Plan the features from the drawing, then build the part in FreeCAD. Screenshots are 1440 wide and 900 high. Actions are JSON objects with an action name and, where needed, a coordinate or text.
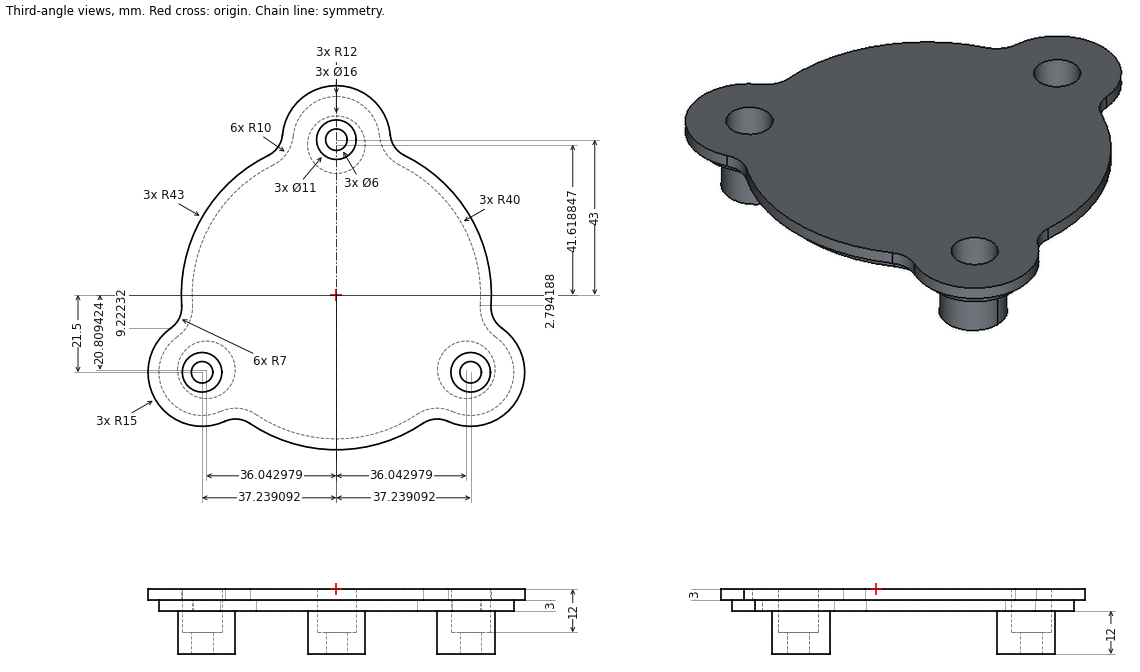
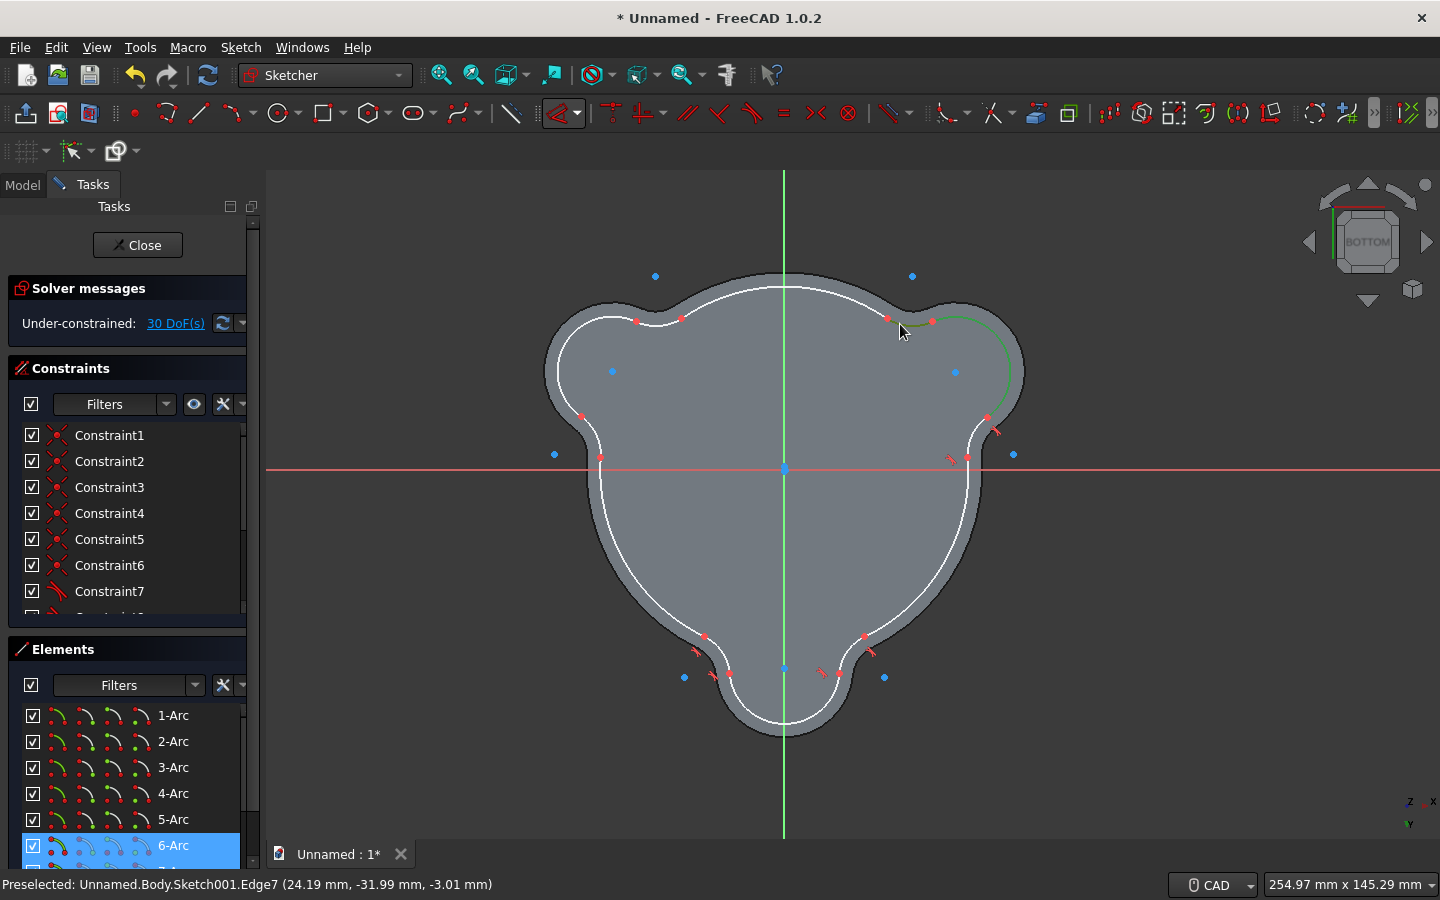
{"action": "left_click", "coordinate": [752, 114]}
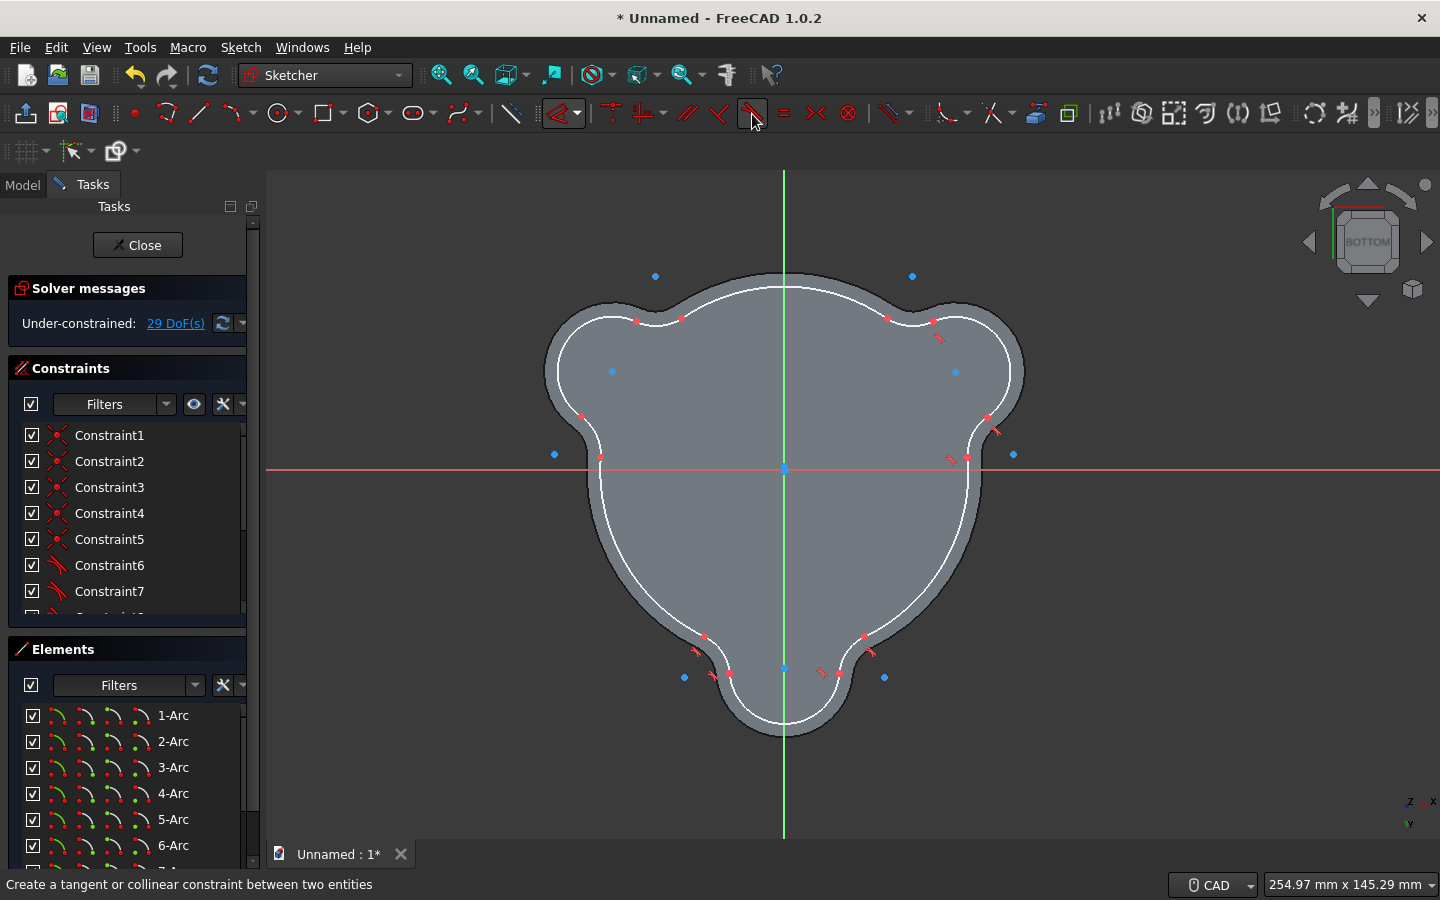
{"action": "left_click", "coordinate": [900, 324]}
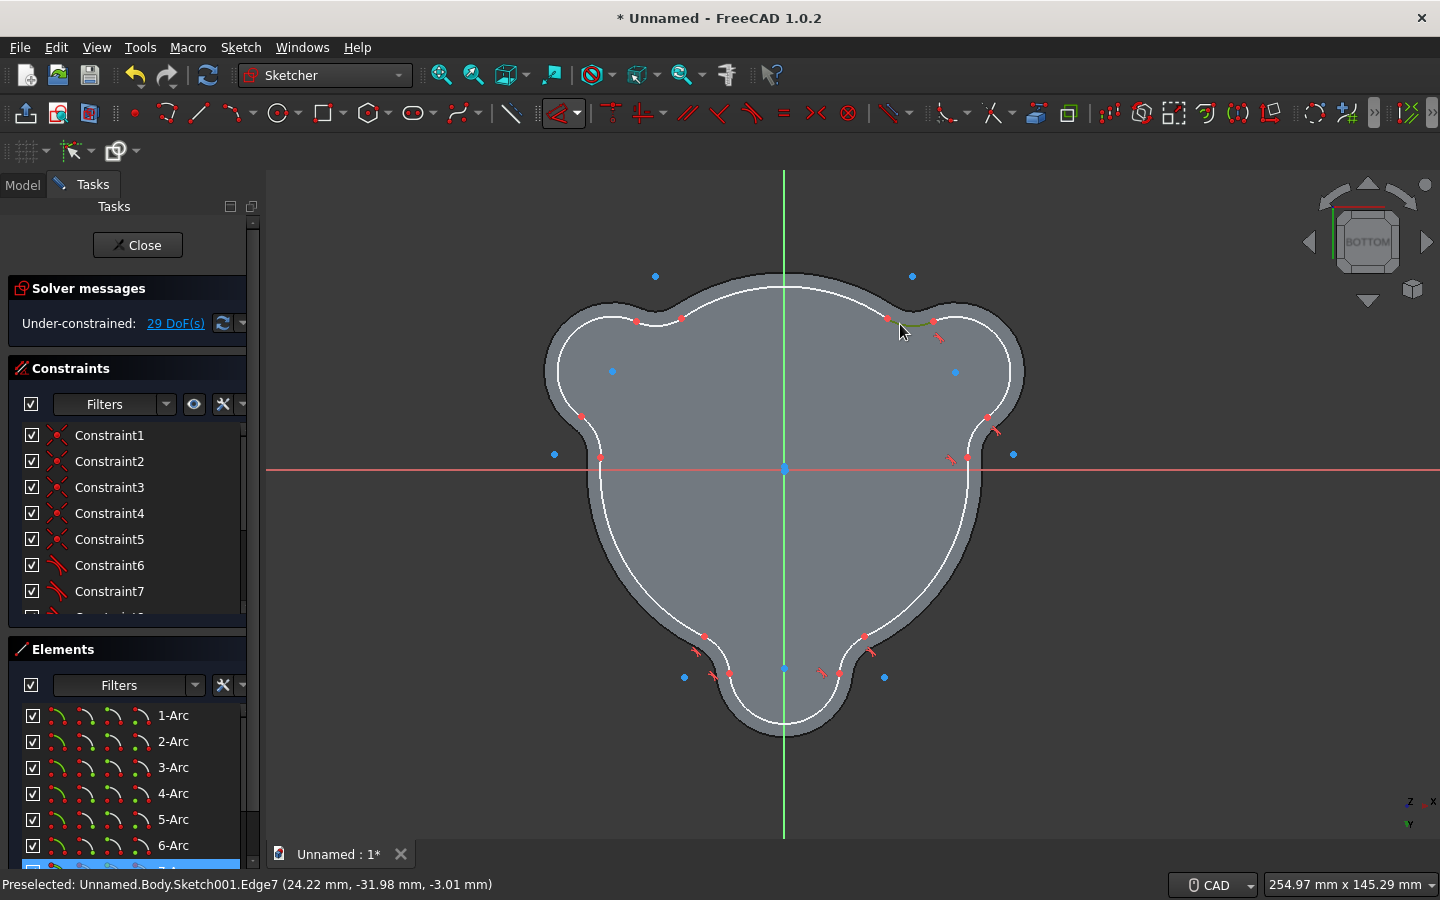
{"action": "left_click", "coordinate": [828, 292]}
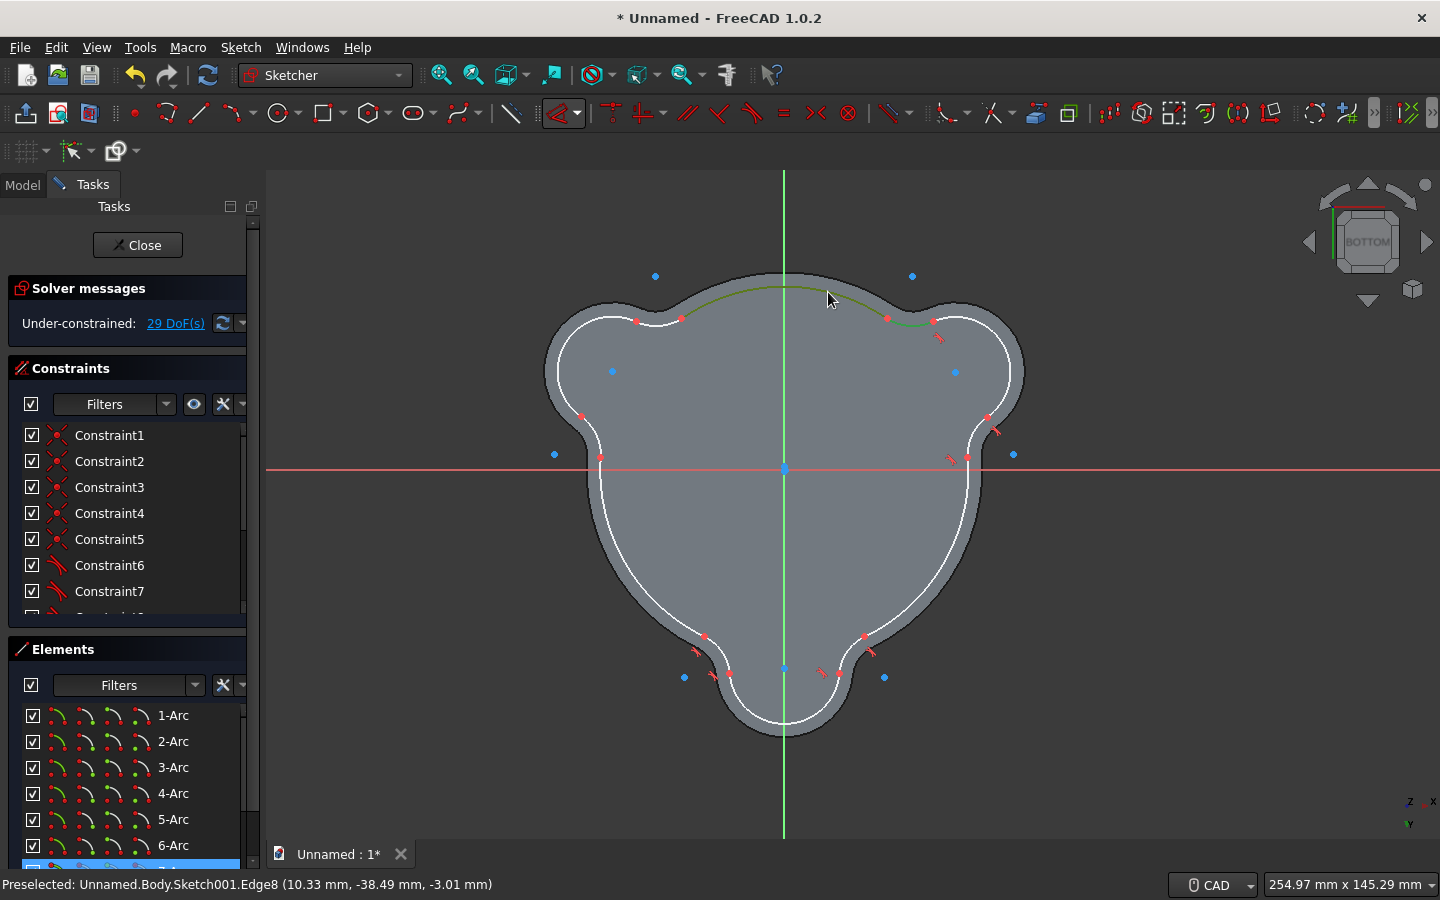
{"action": "left_click", "coordinate": [752, 114]}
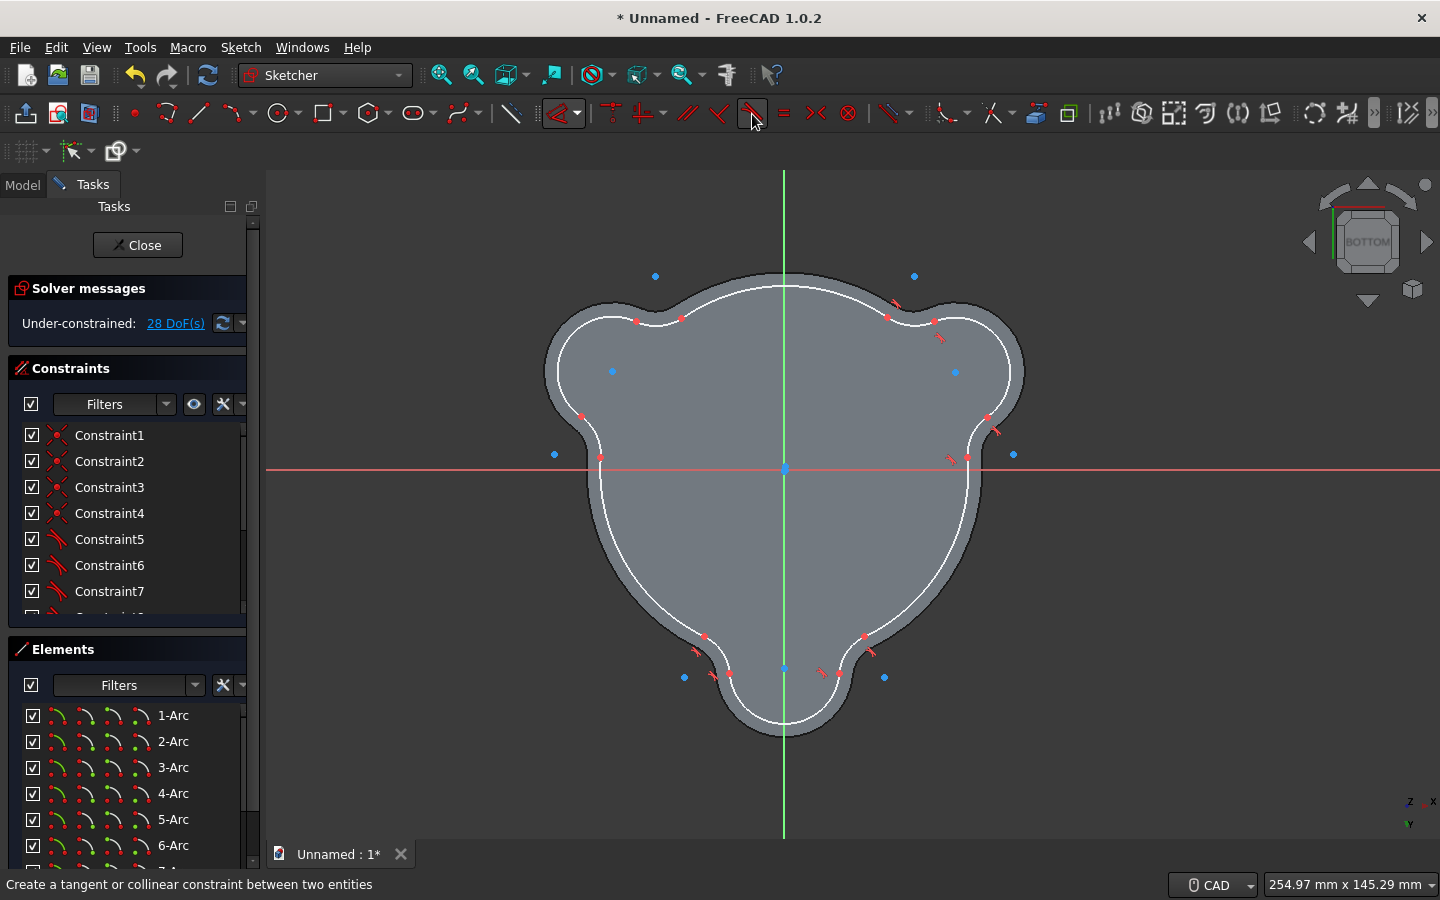
{"action": "left_click", "coordinate": [827, 291]}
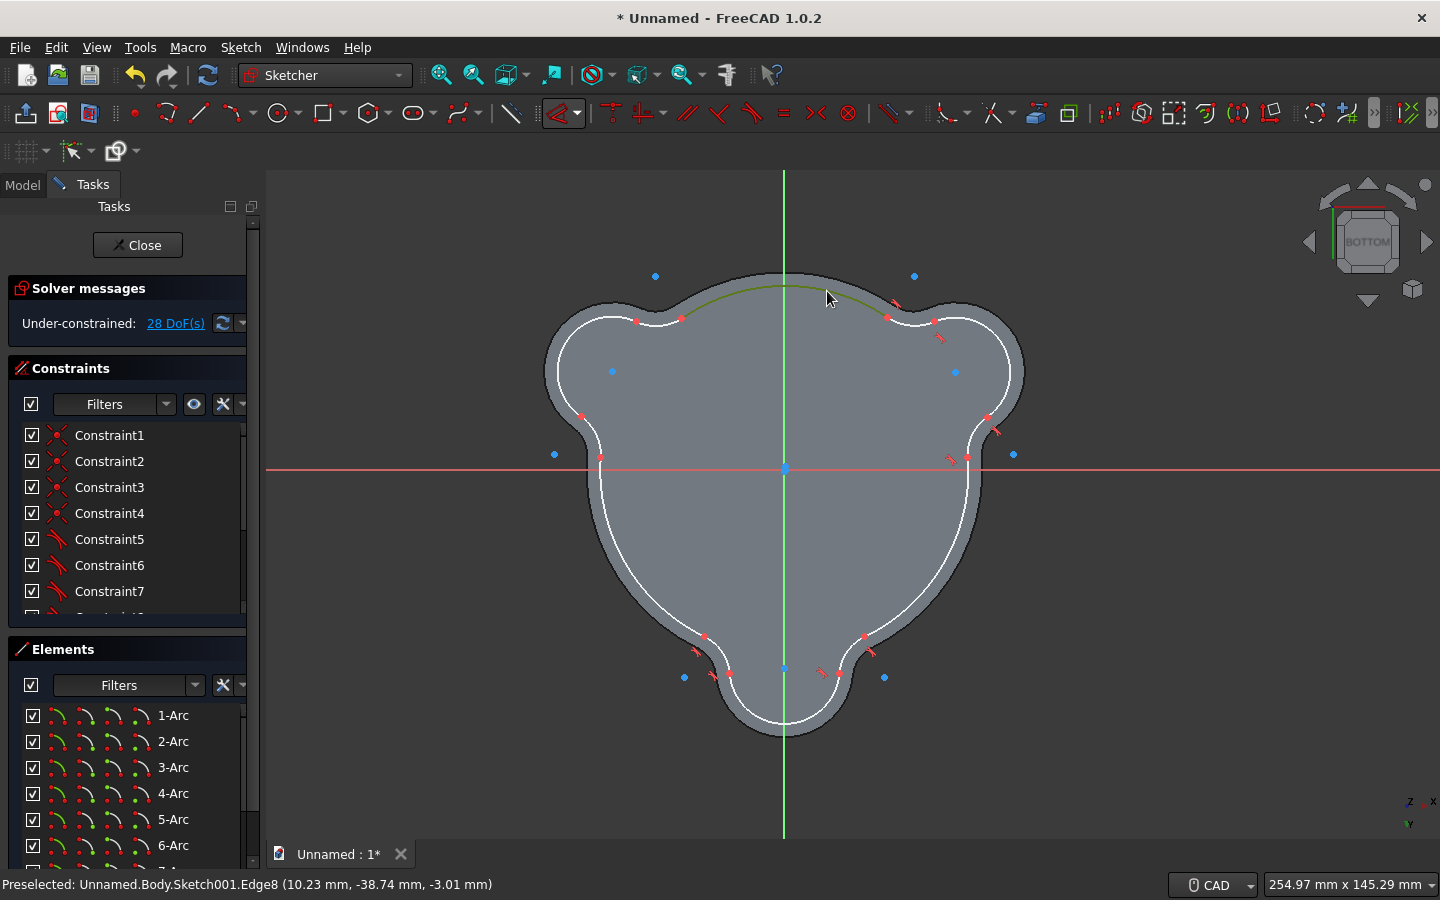
{"action": "left_click", "coordinate": [650, 326]}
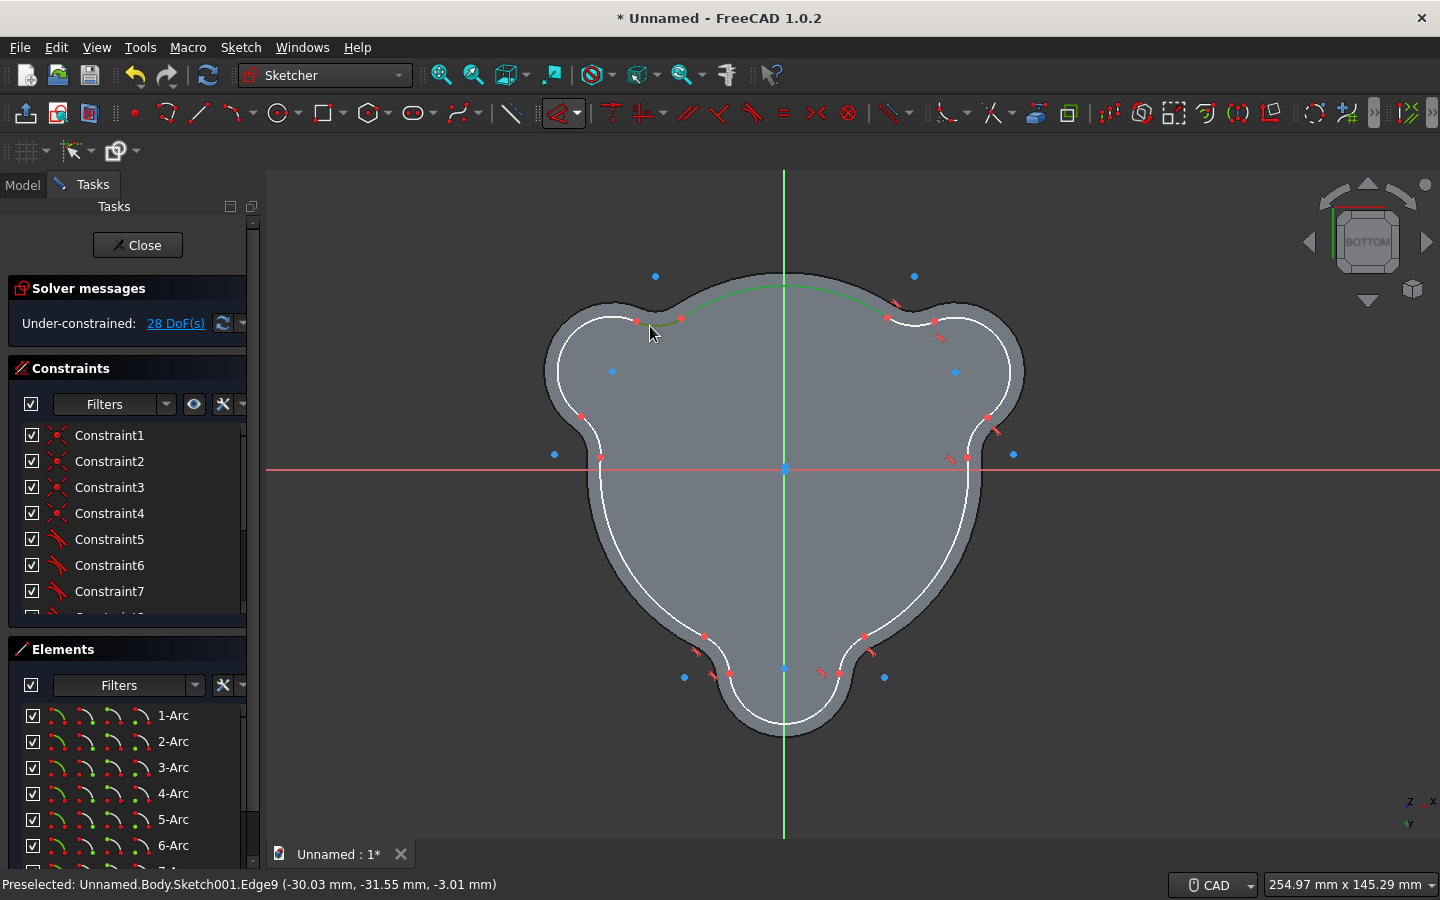
{"action": "left_click", "coordinate": [752, 114]}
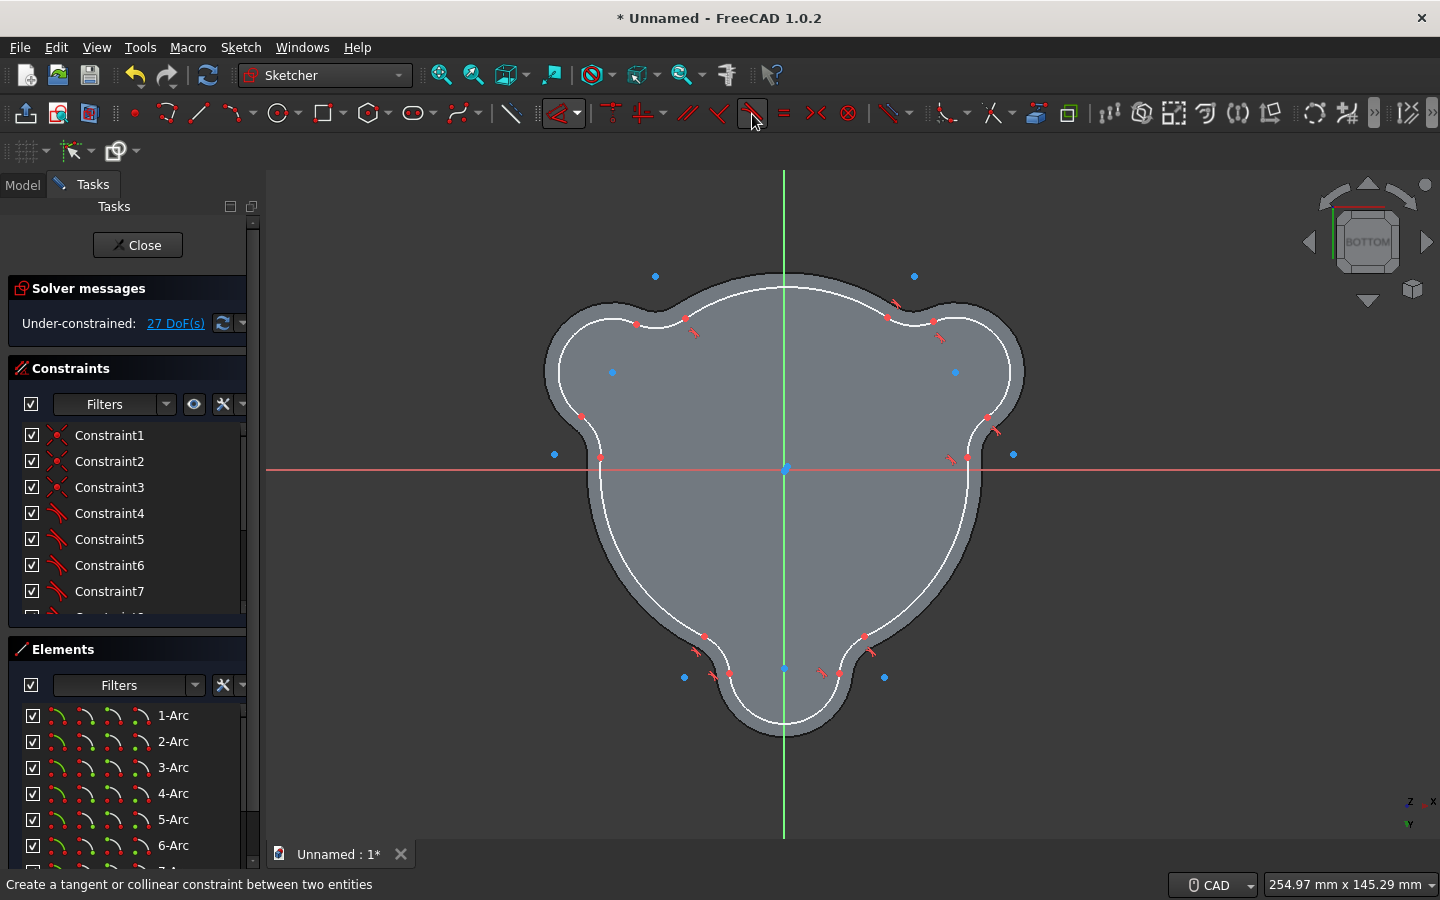
{"action": "left_click", "coordinate": [651, 328]}